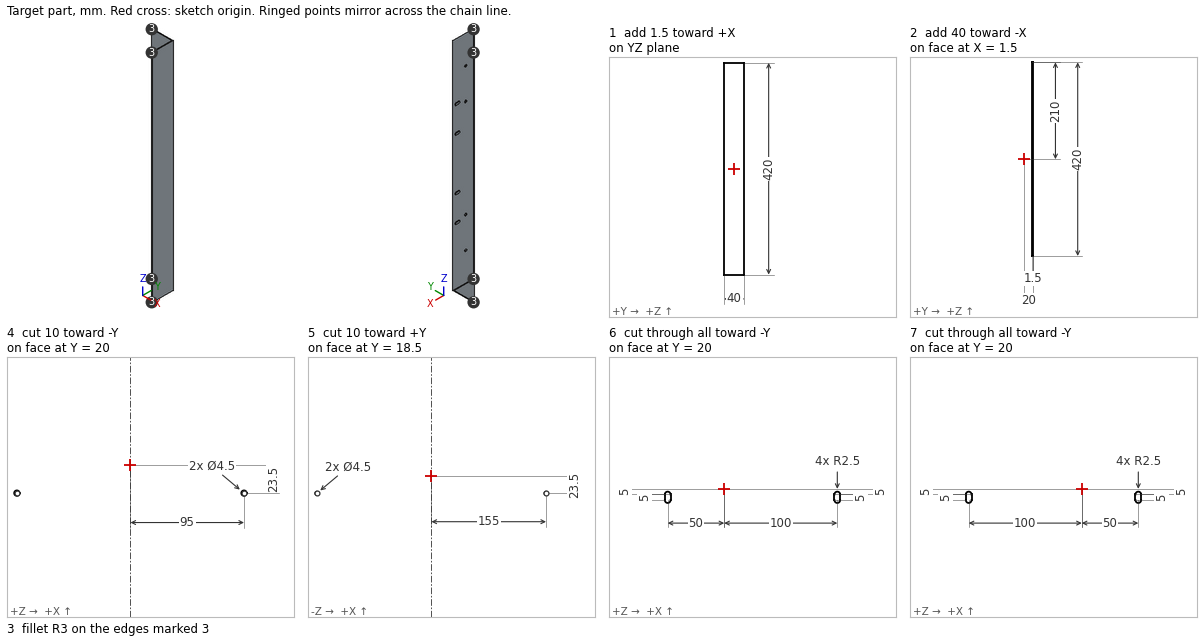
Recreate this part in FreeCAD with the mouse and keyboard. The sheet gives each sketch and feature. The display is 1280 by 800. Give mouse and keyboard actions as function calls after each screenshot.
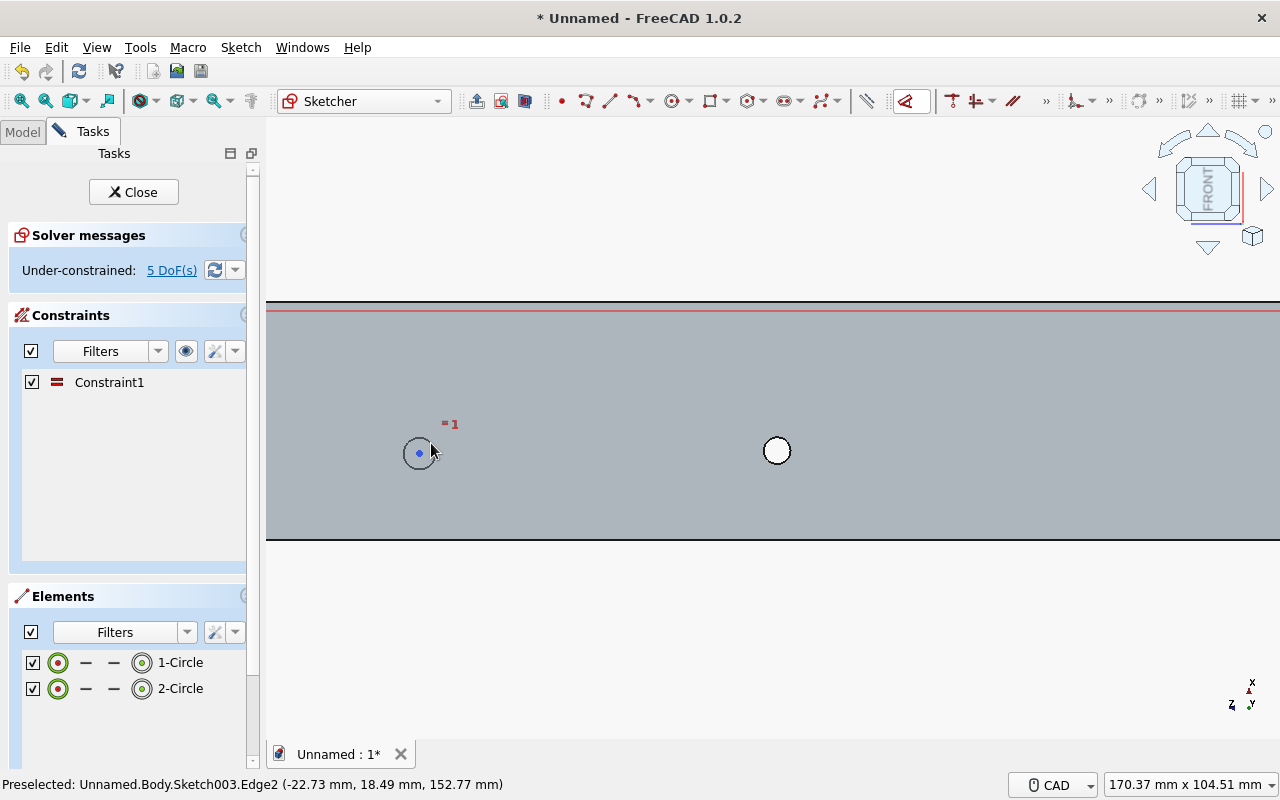
scroll(429, 445, down, 6)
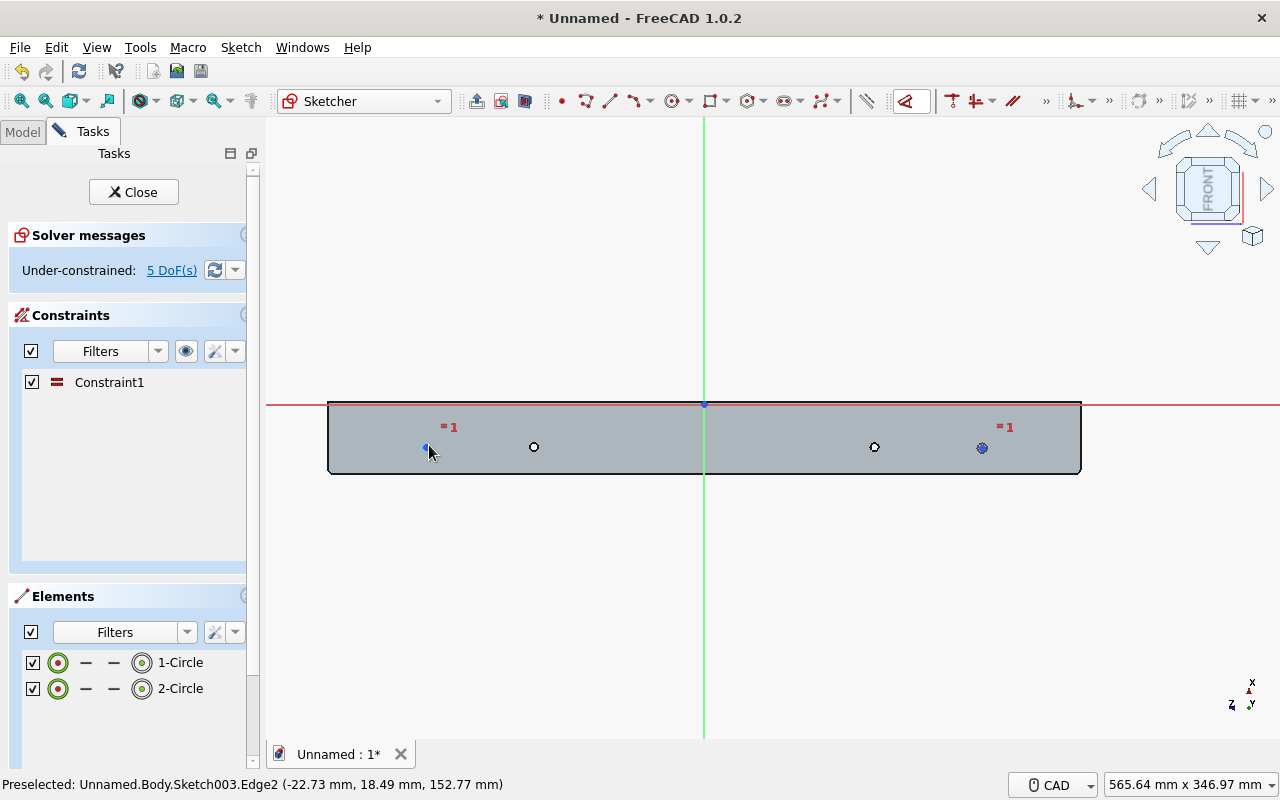
click(982, 448)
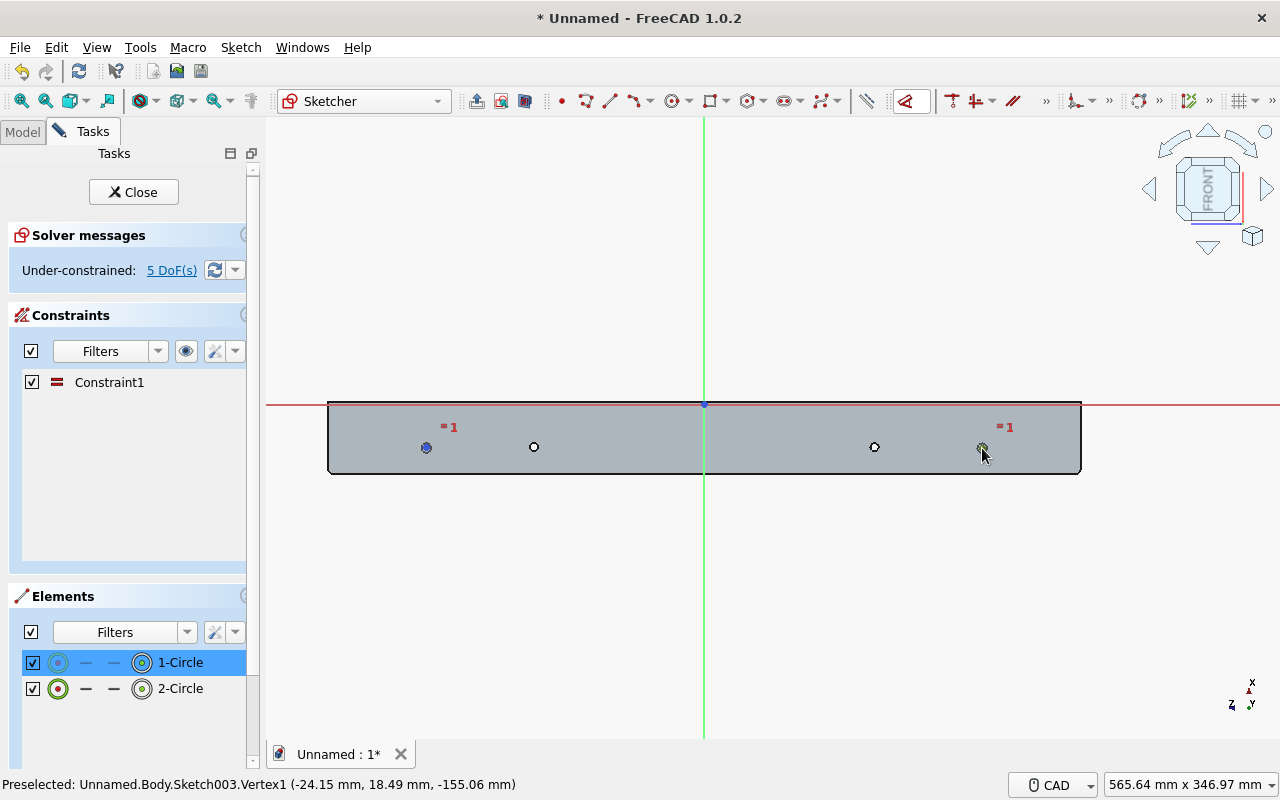
click(426, 448)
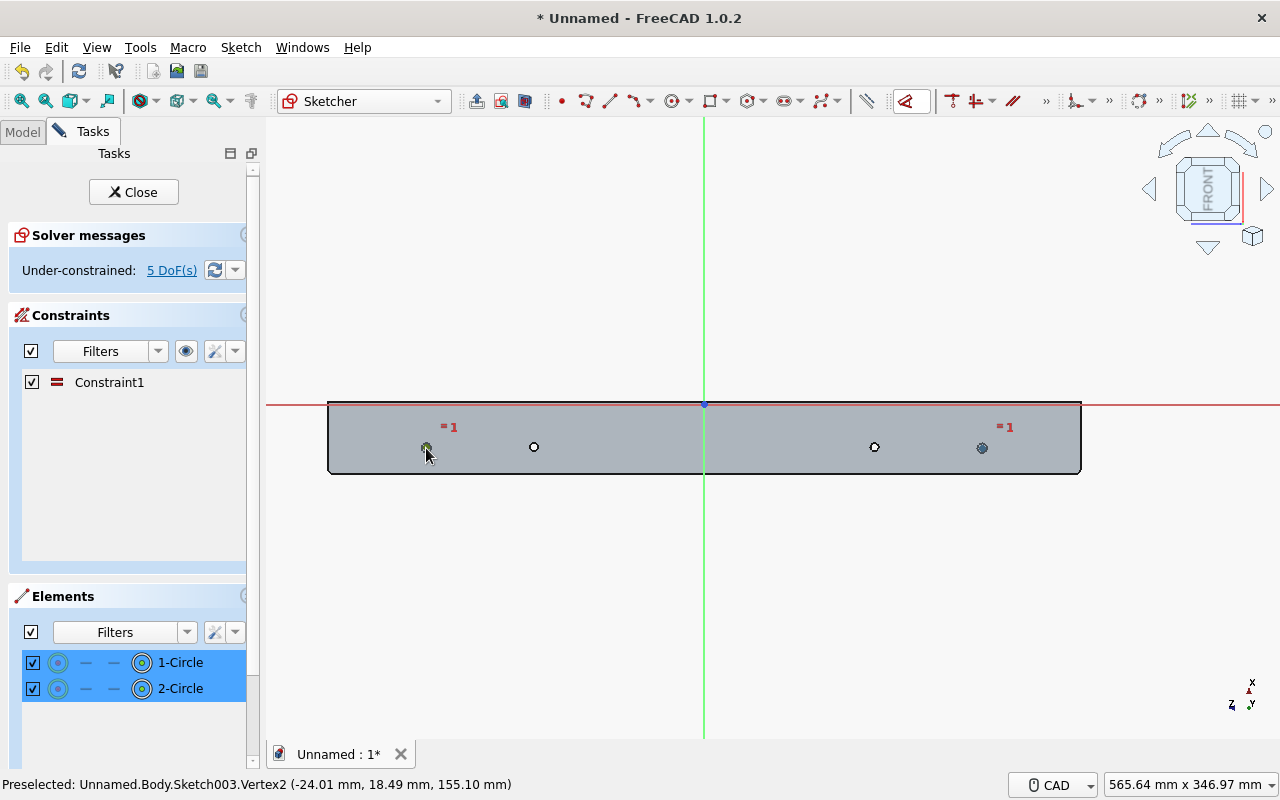
click(704, 671)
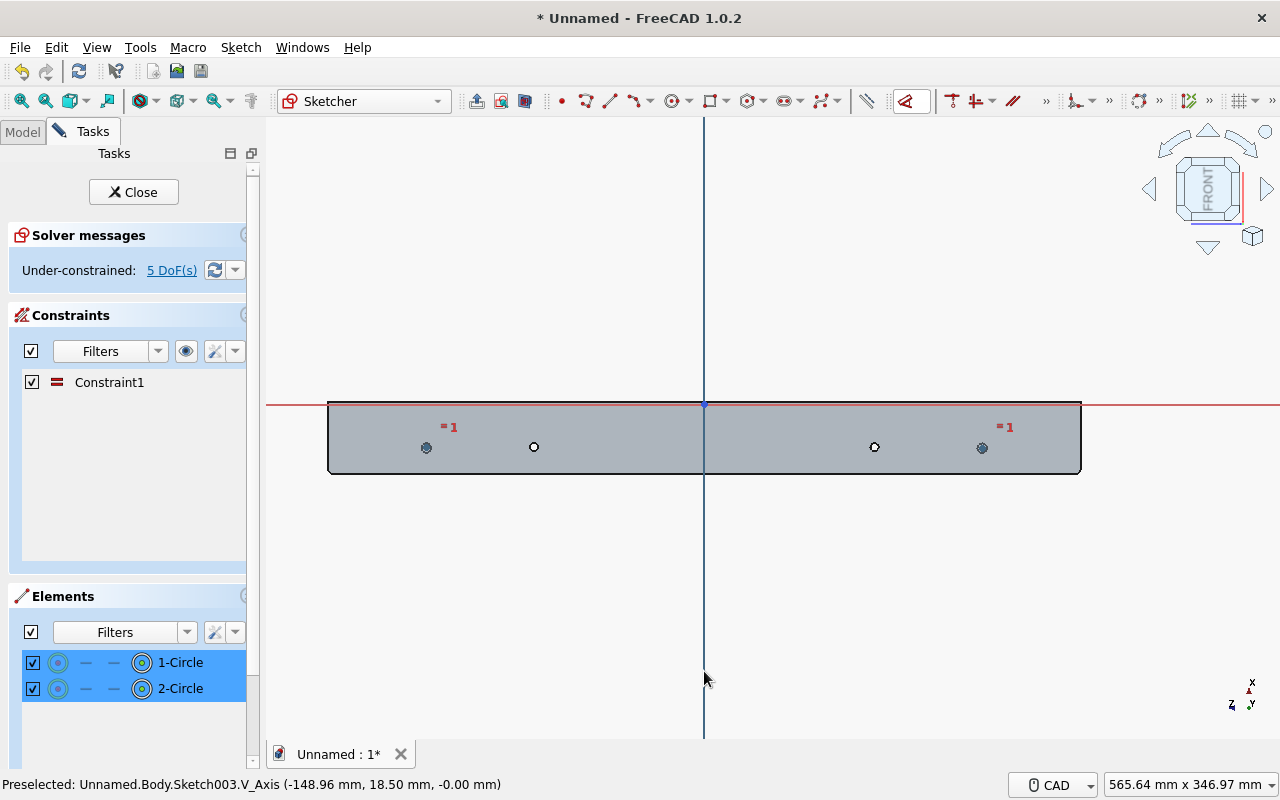
key(s)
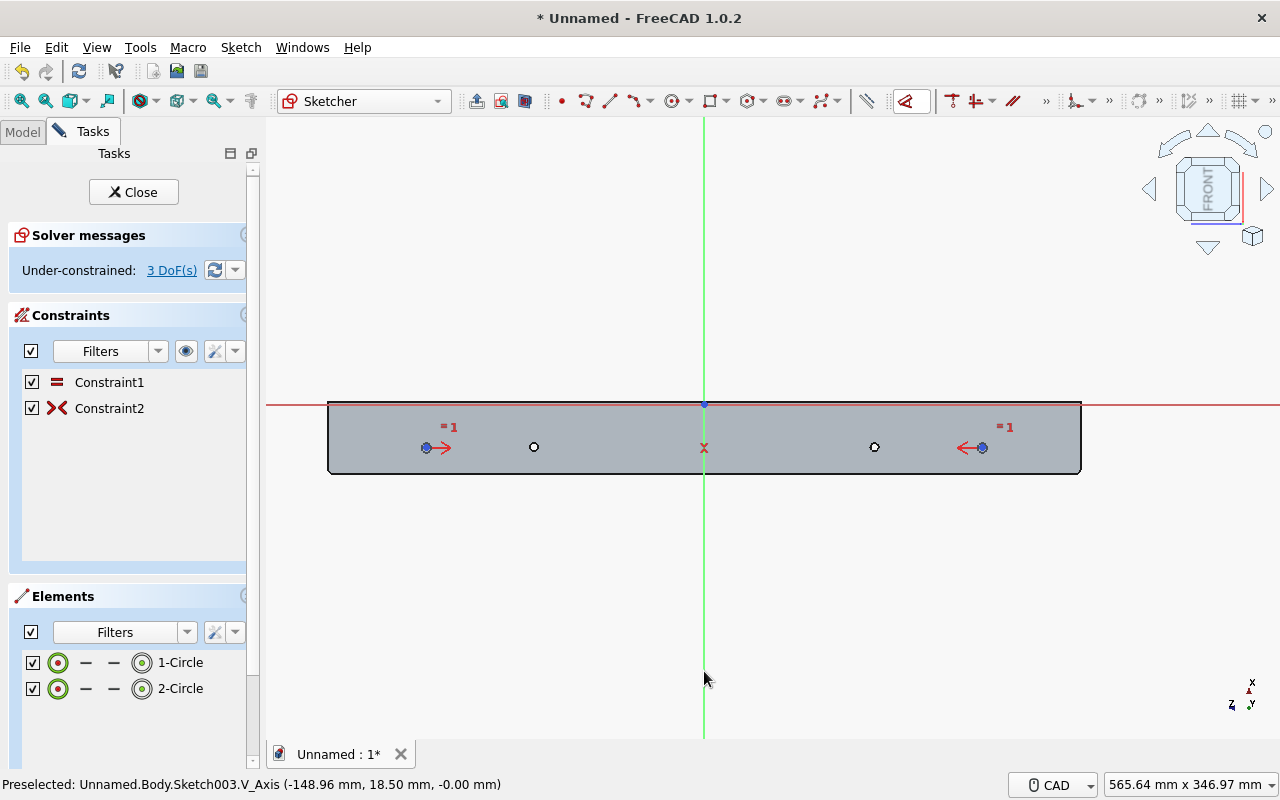
scroll(986, 445, up, 8)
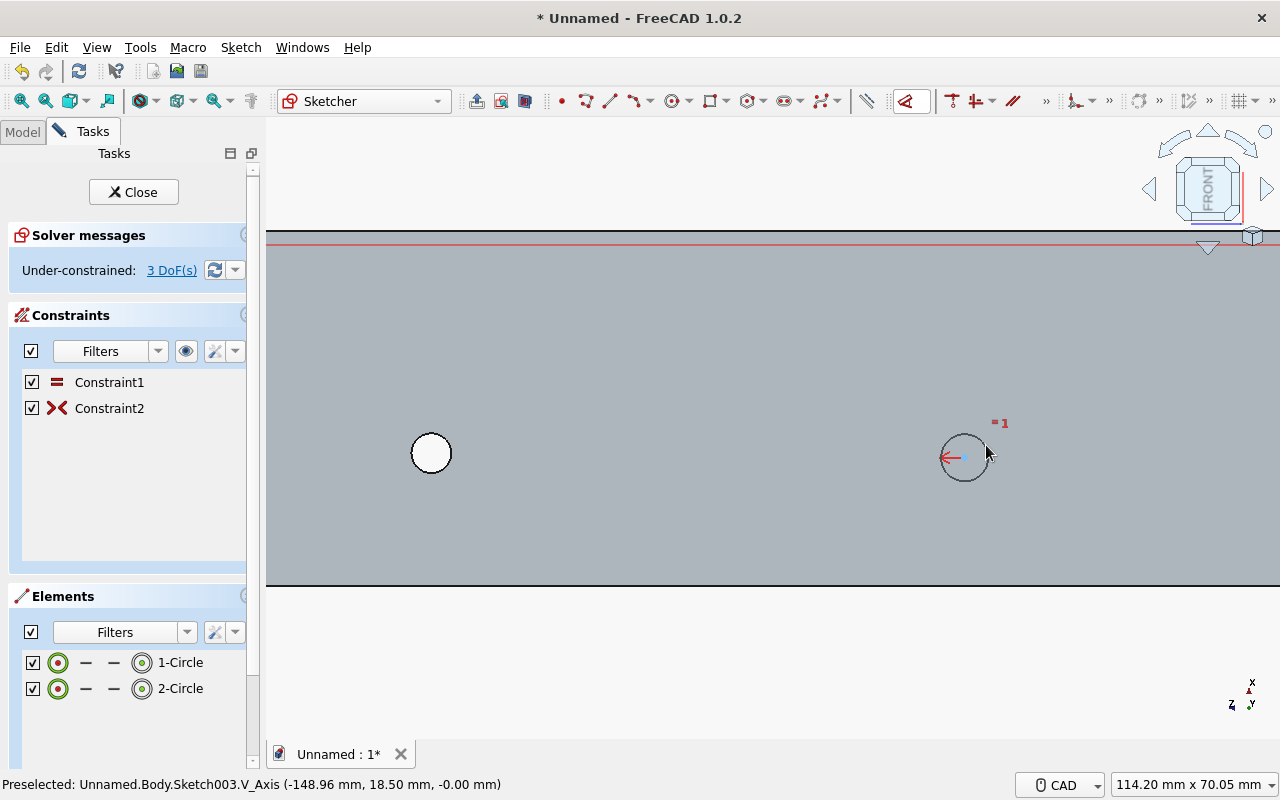
click(981, 441)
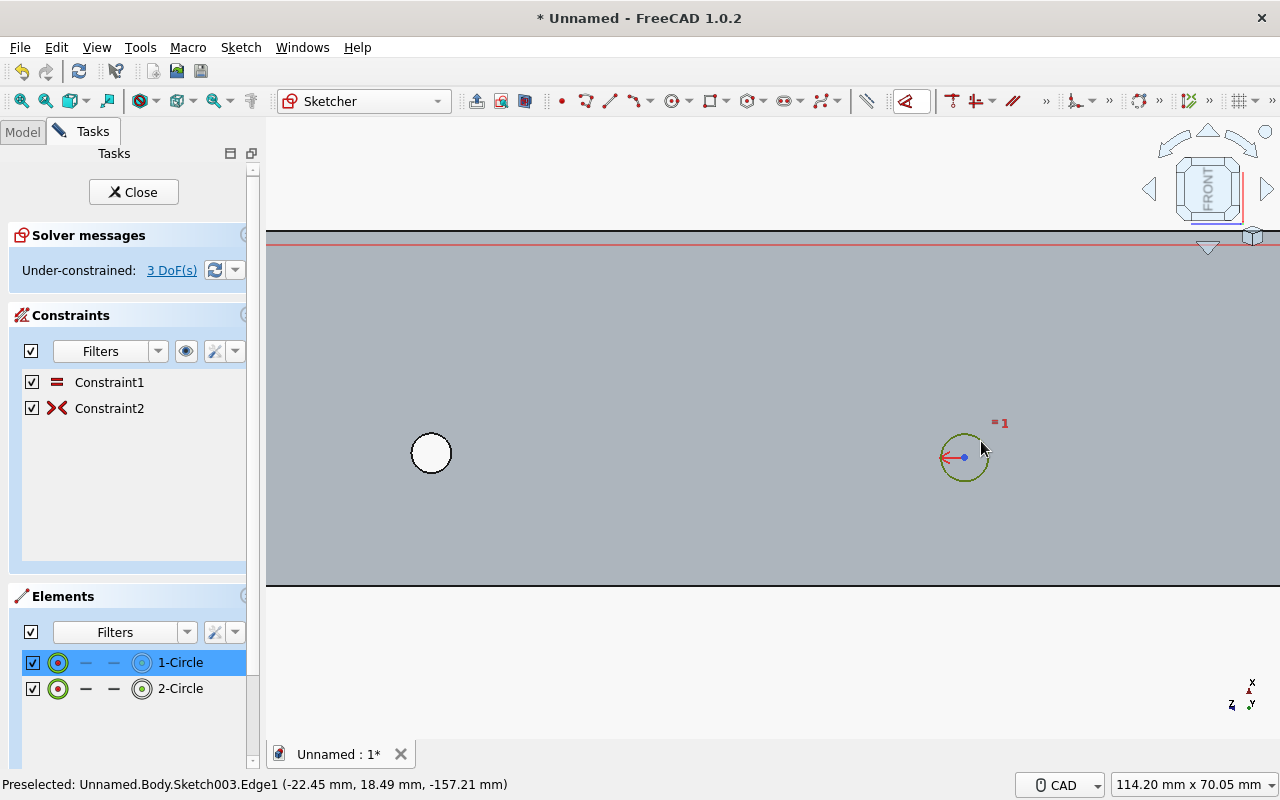
click(924, 102)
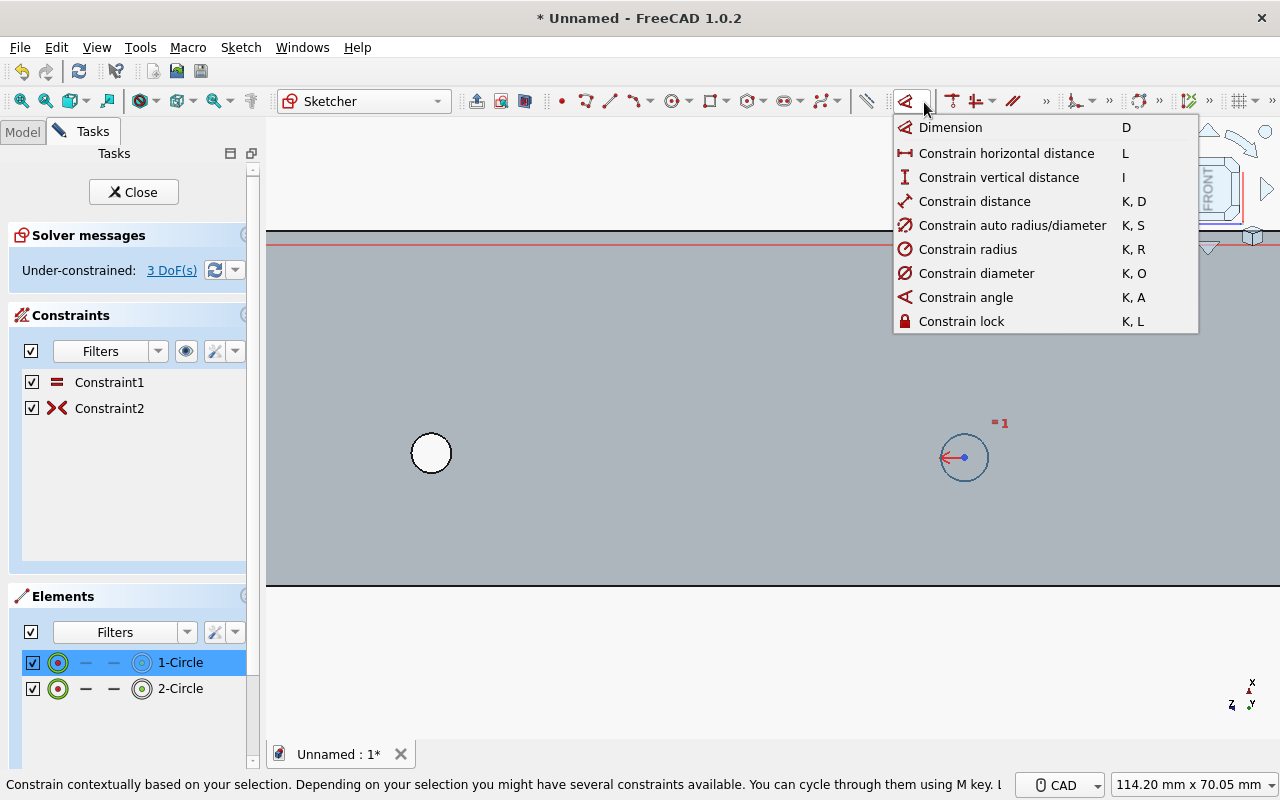
click(1046, 273)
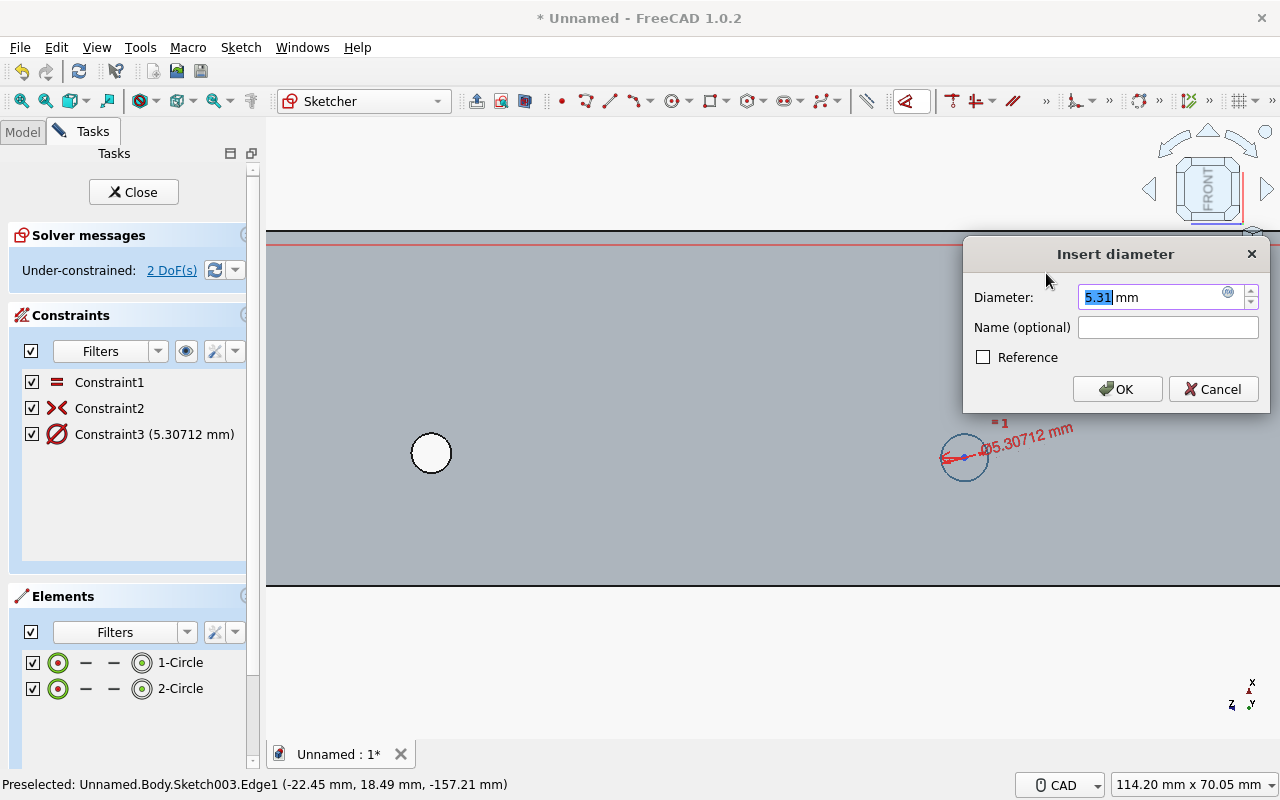
text(4.5)
key(Return)